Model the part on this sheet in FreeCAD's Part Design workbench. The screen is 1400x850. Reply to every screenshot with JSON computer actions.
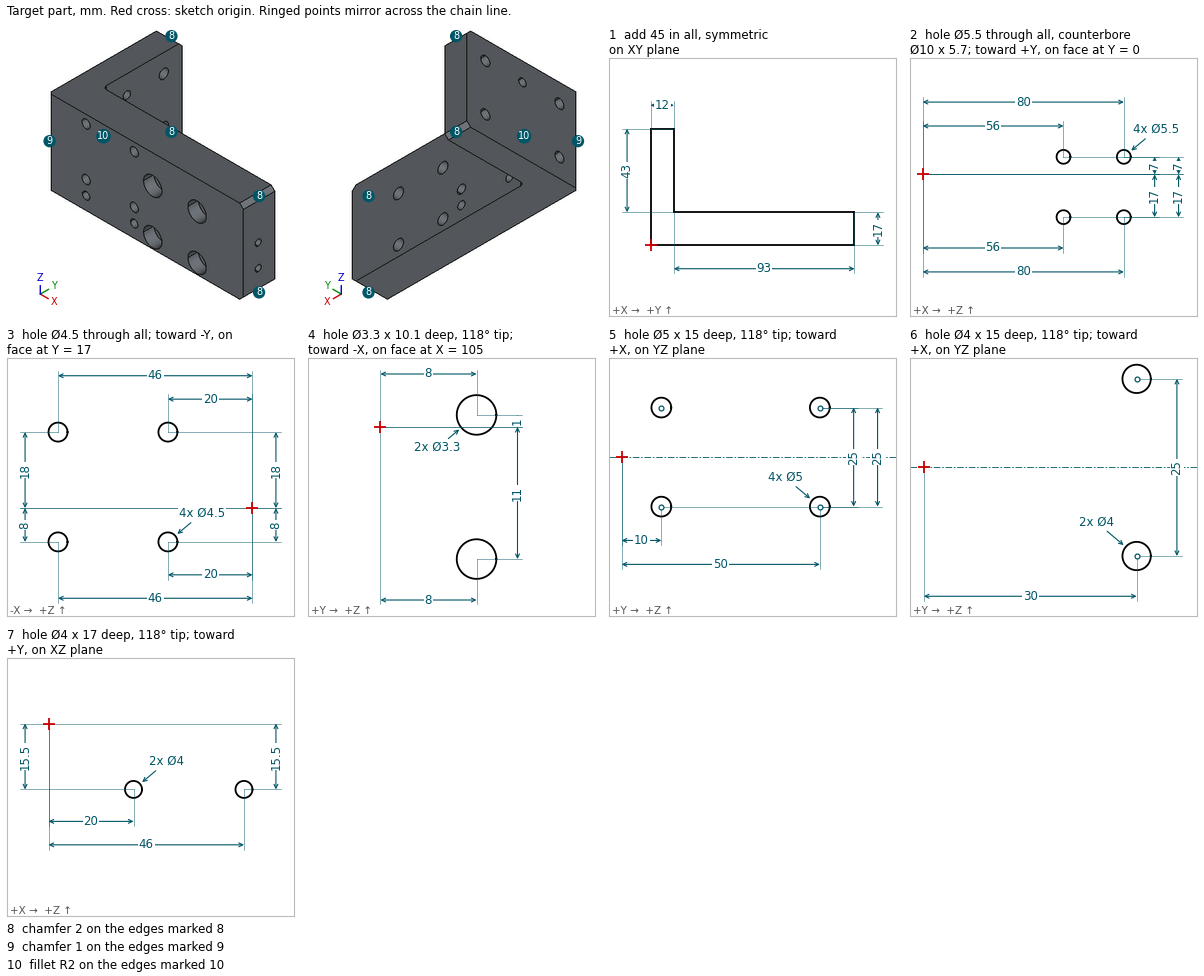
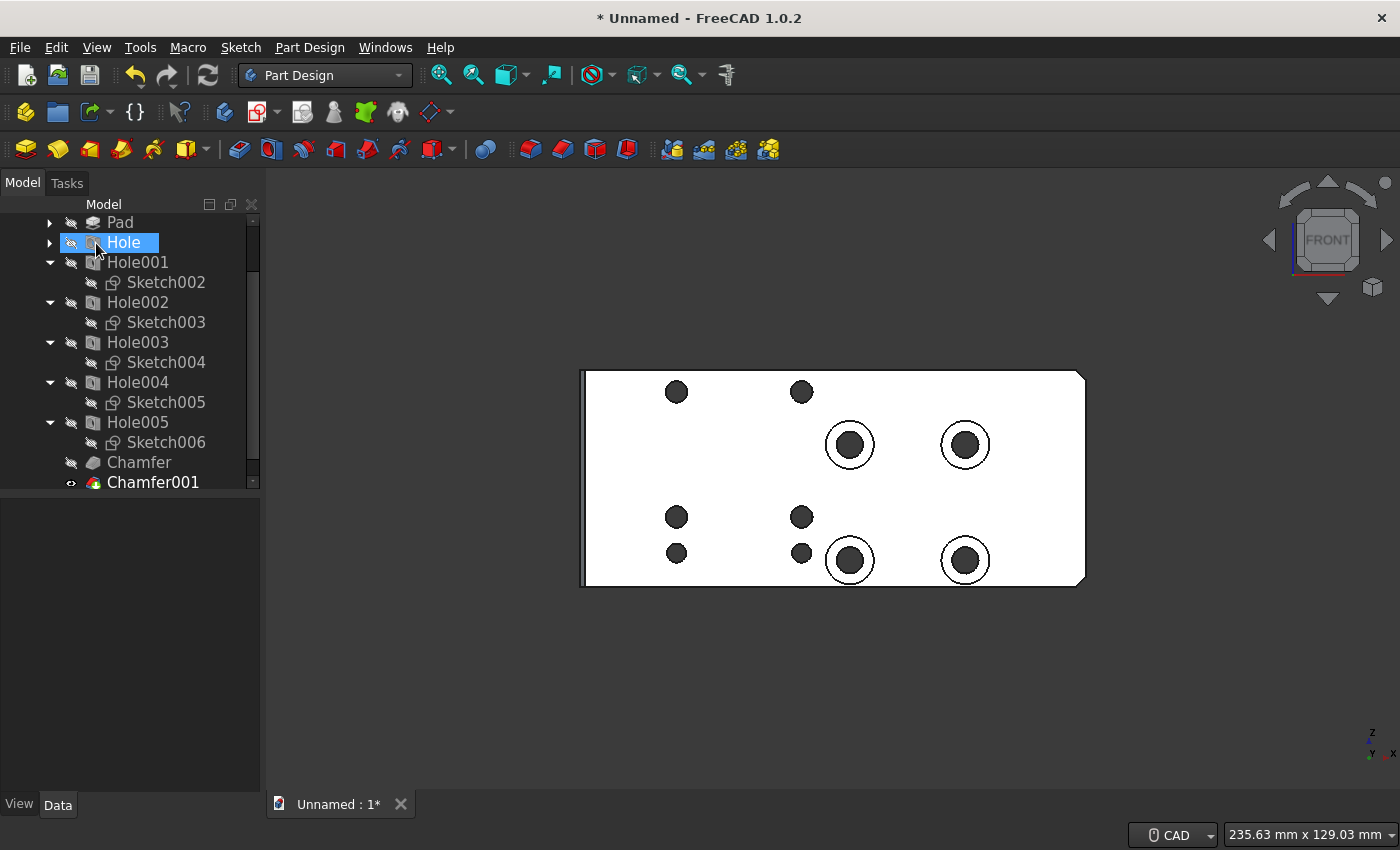
{"action": "key", "text": "0"}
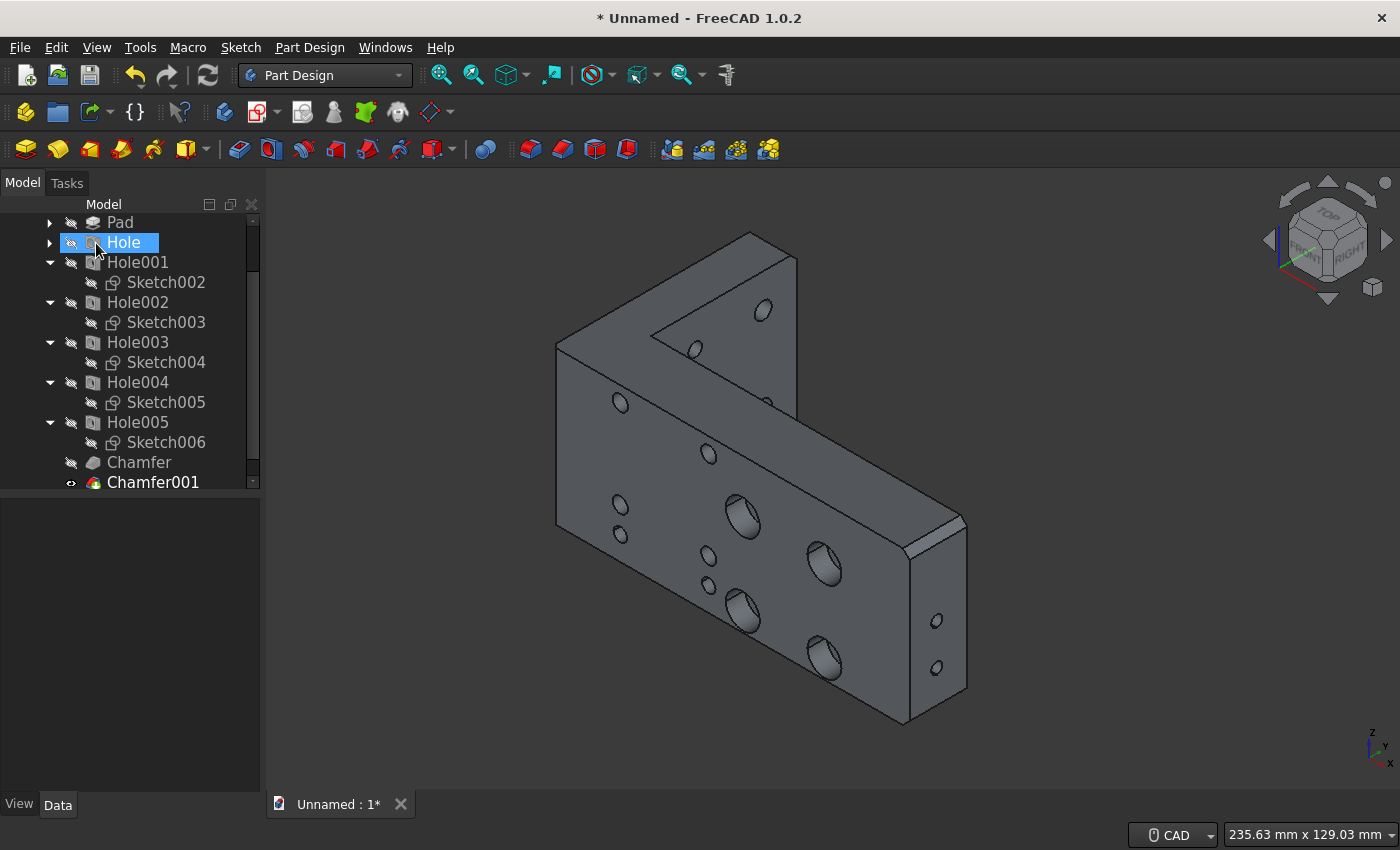
{"action": "key", "text": "2"}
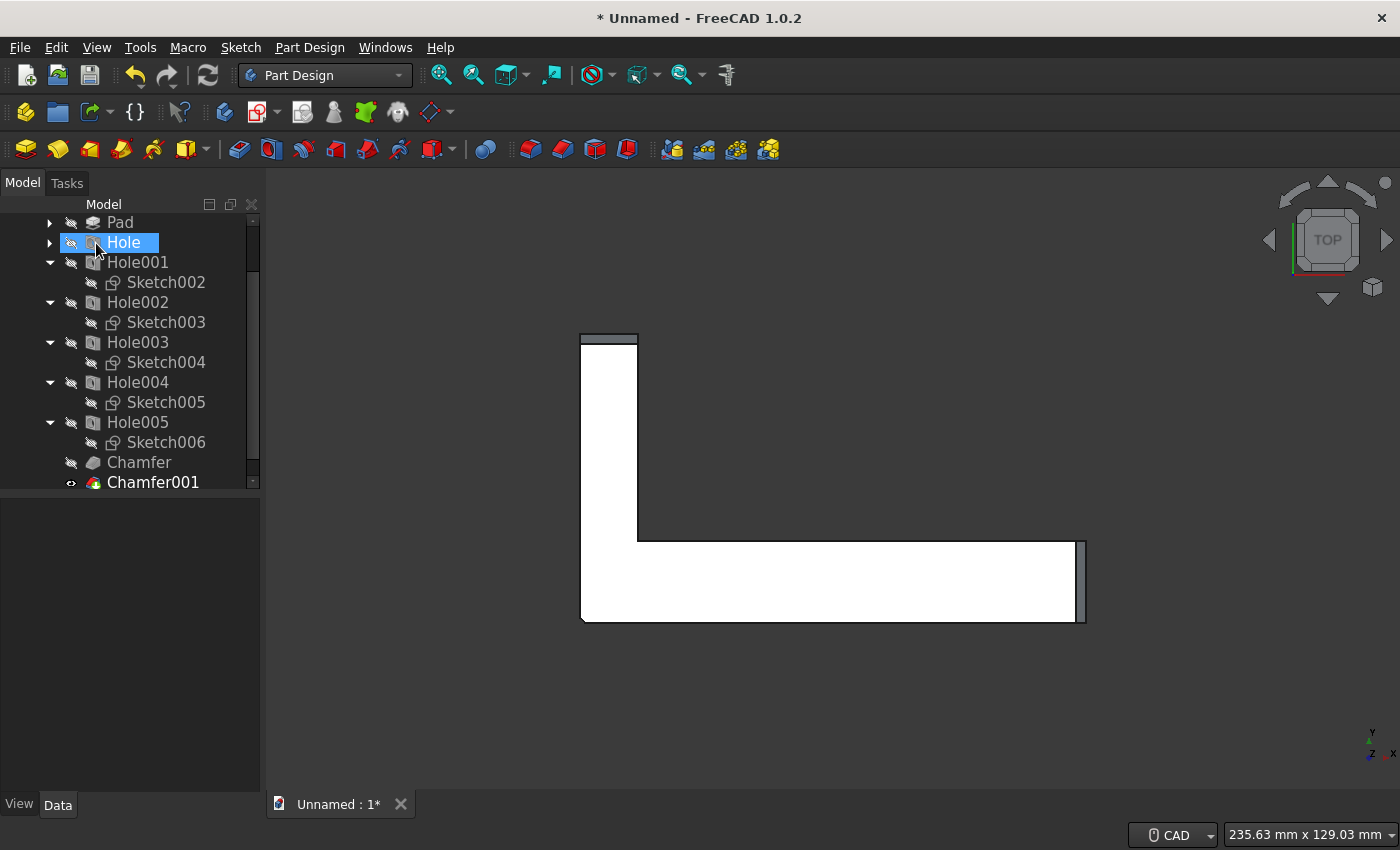
{"action": "key", "text": "1"}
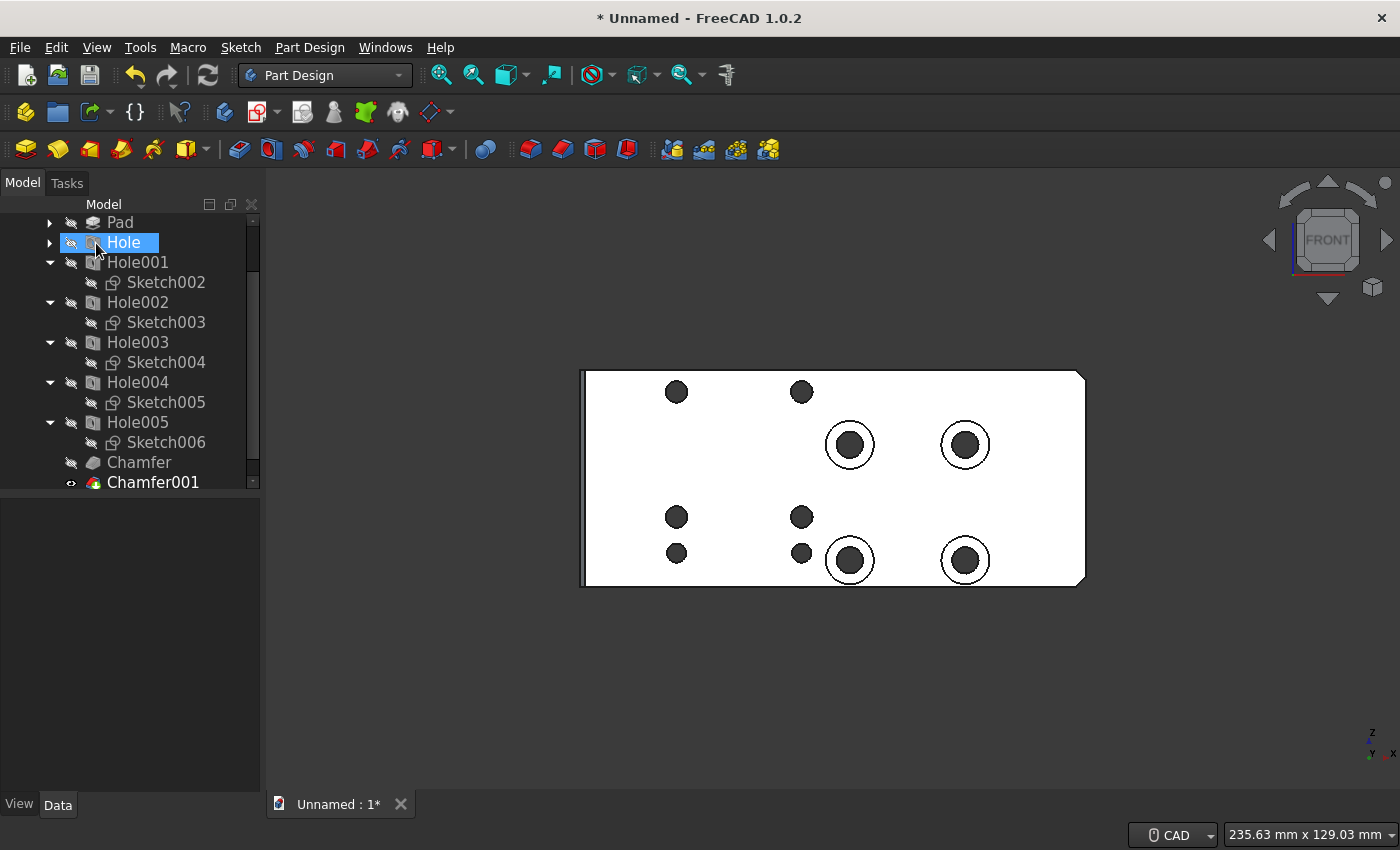
{"action": "left_click", "coordinate": [442, 76]}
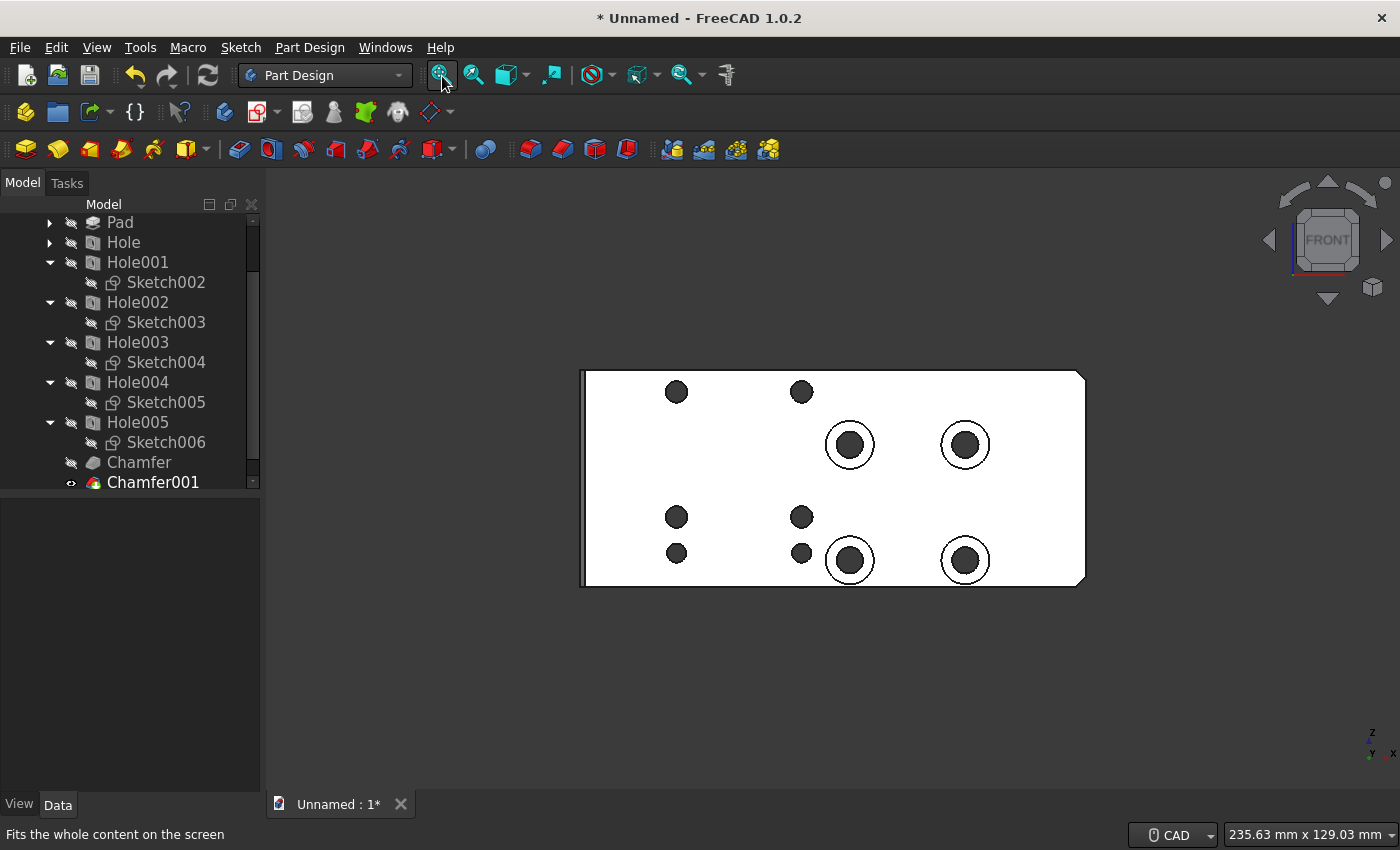
{"action": "key", "text": "3"}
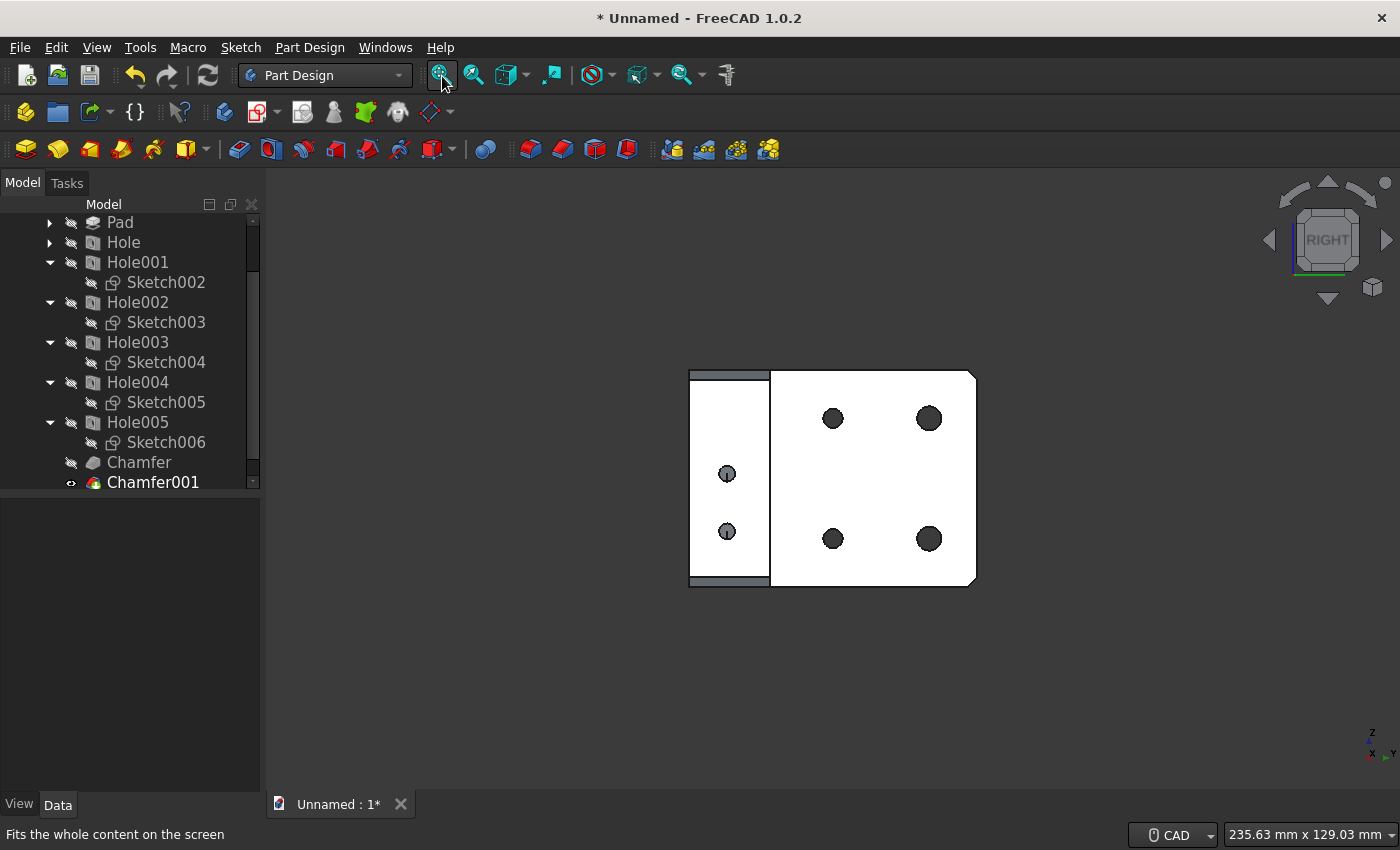
{"action": "key", "text": "v f"}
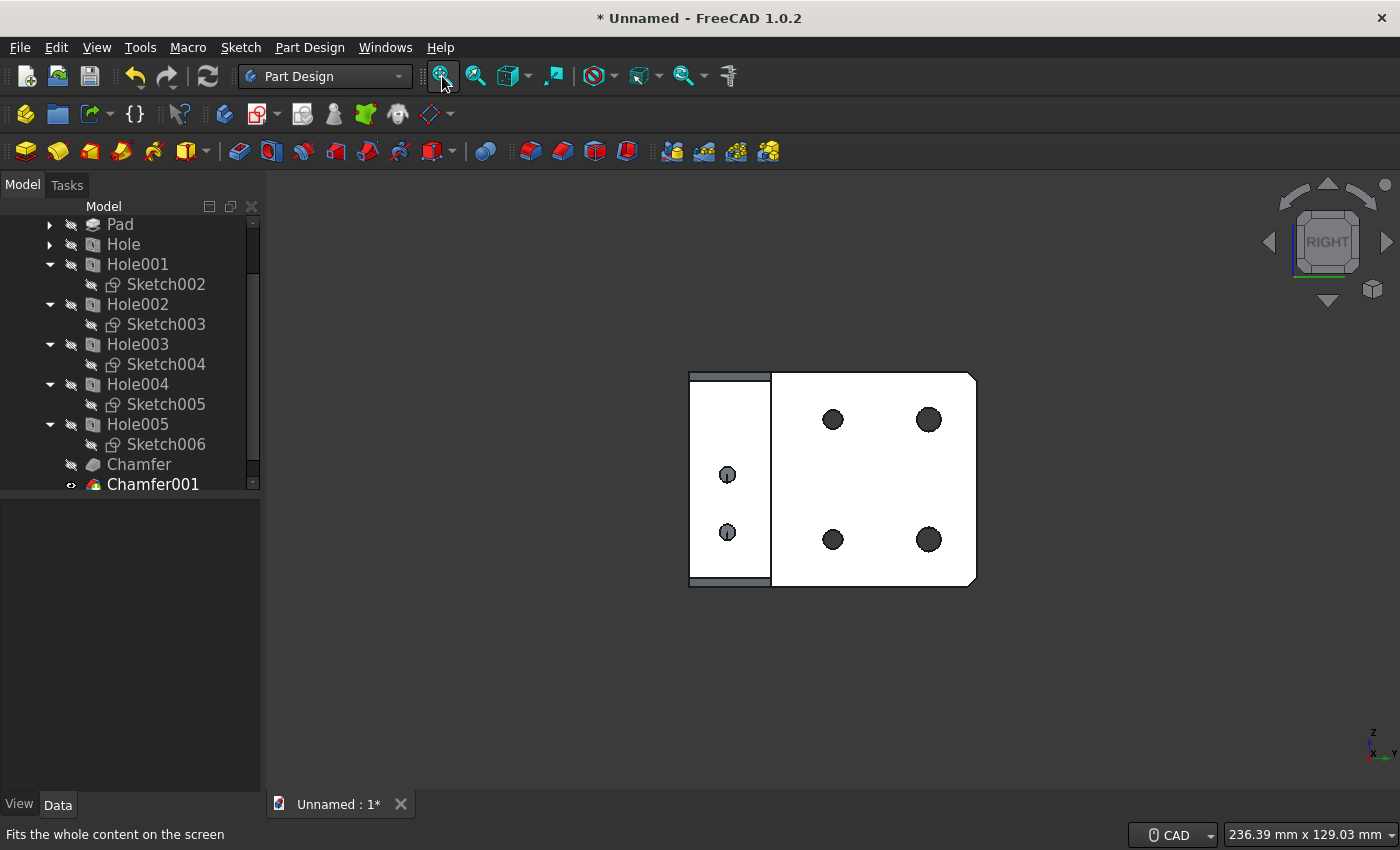
{"action": "key", "text": "5"}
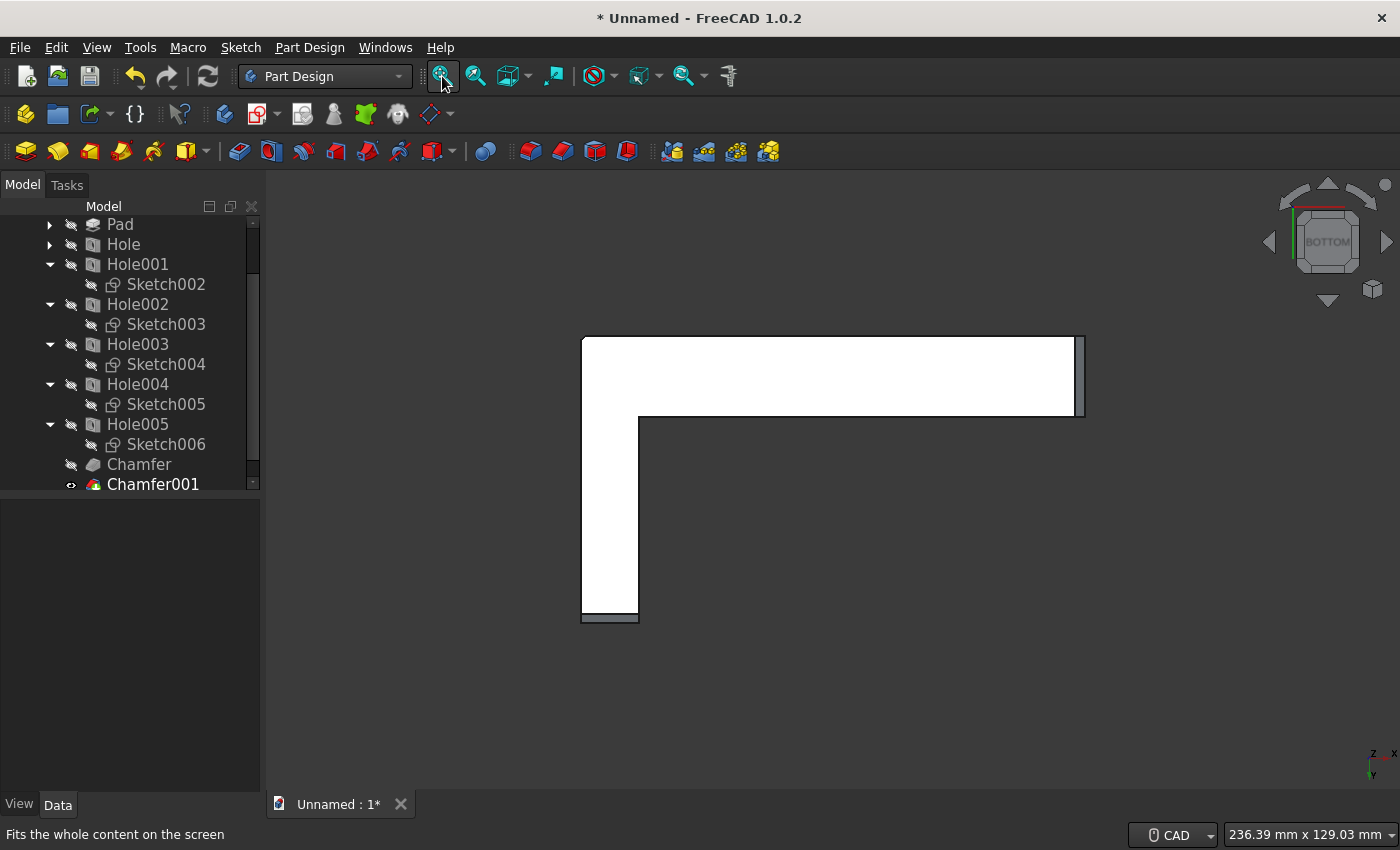
{"action": "key", "text": "4"}